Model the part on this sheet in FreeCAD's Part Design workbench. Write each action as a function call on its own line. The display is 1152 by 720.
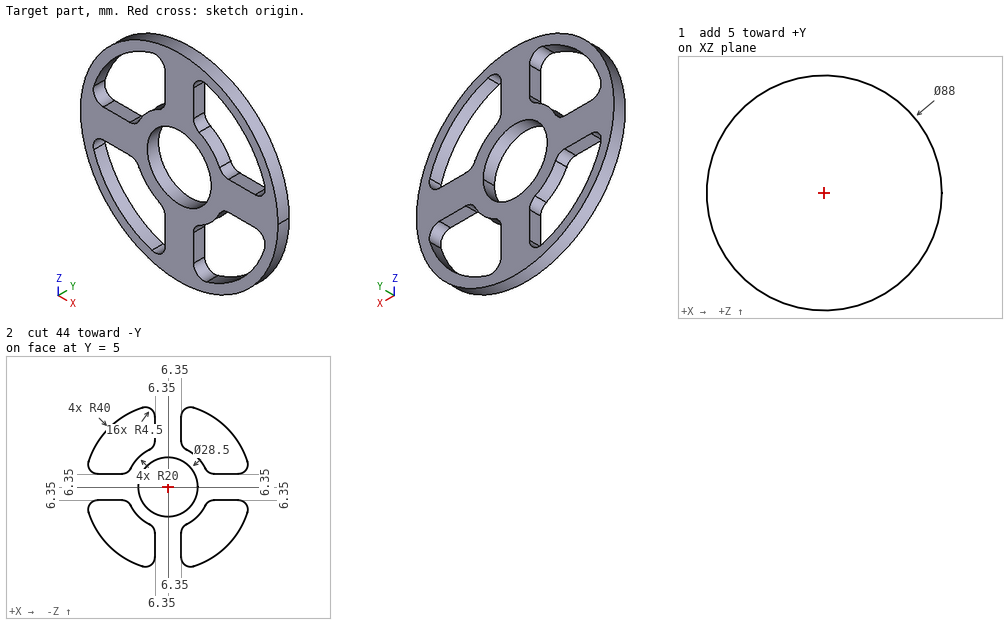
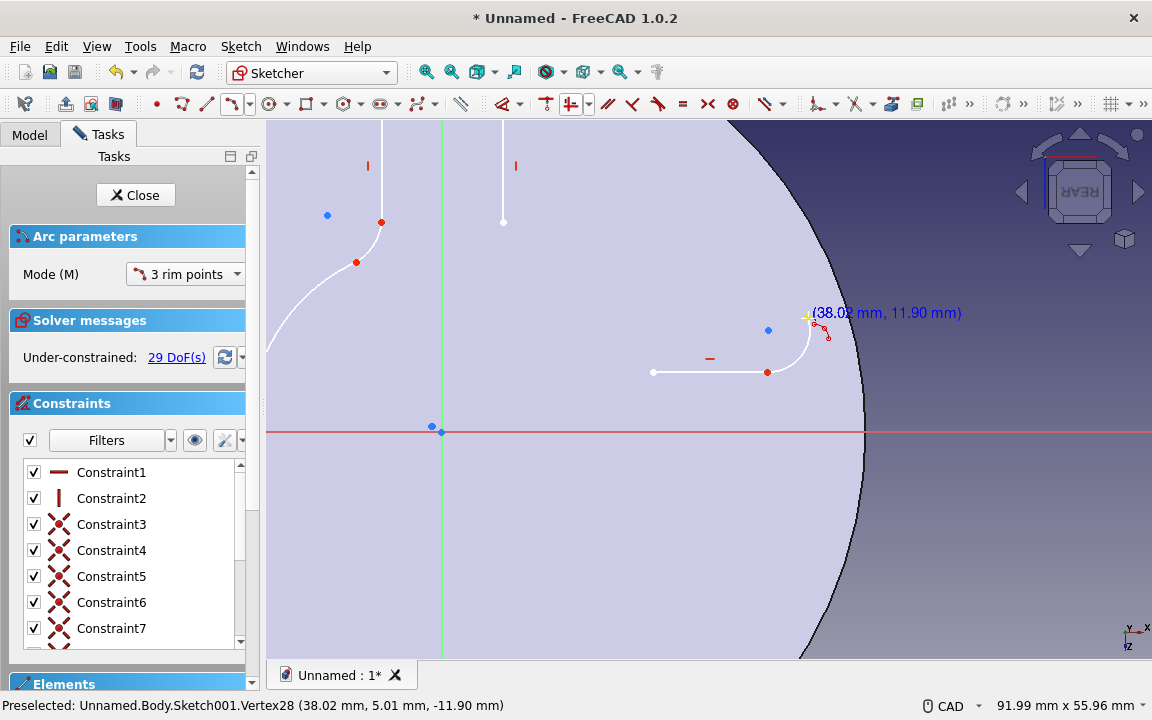
scroll(803, 354, down, 4)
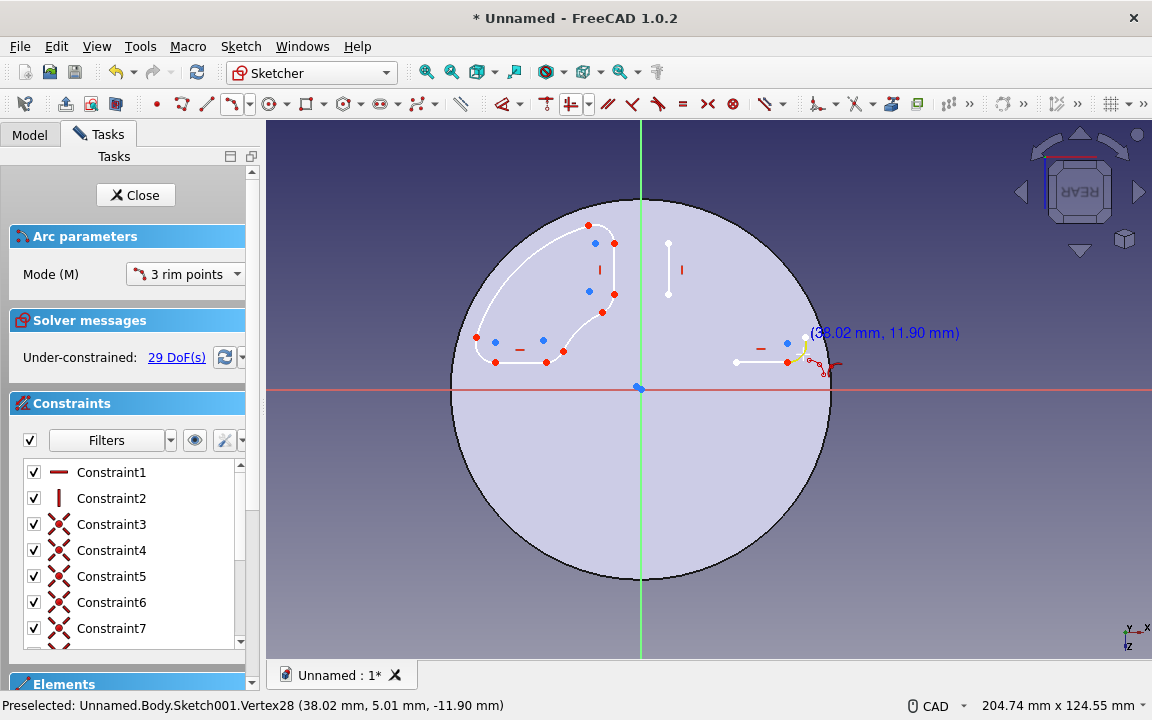
click(694, 225)
click(763, 267)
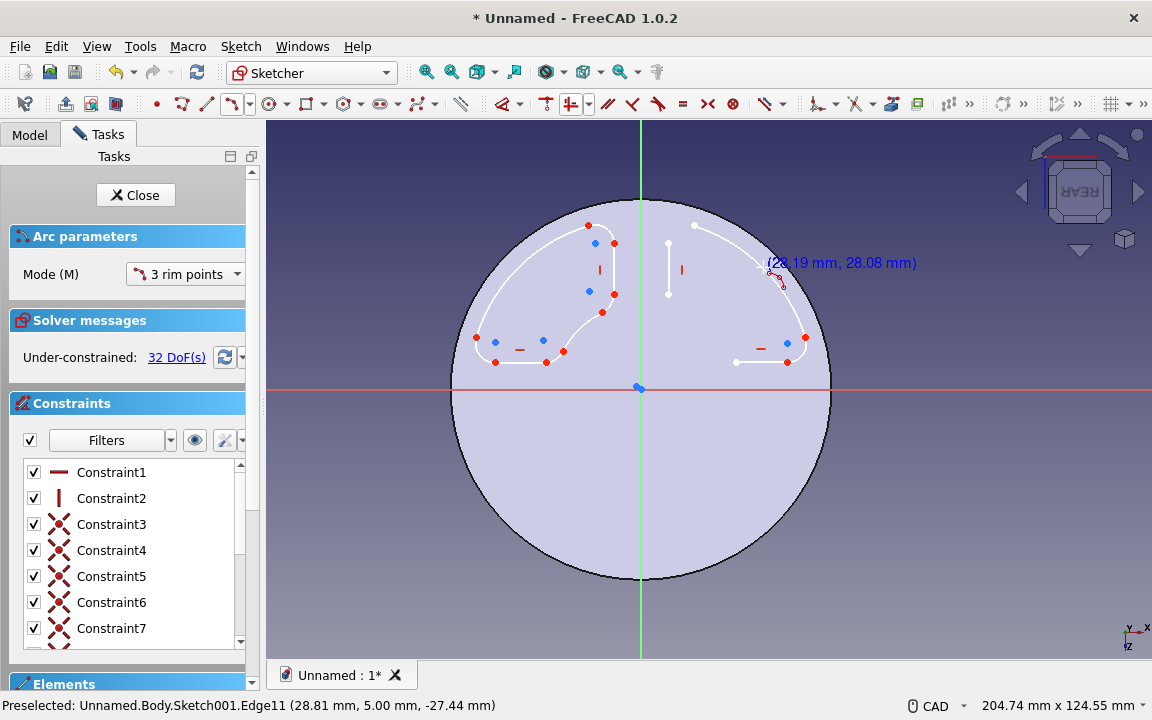
click(694, 226)
click(669, 244)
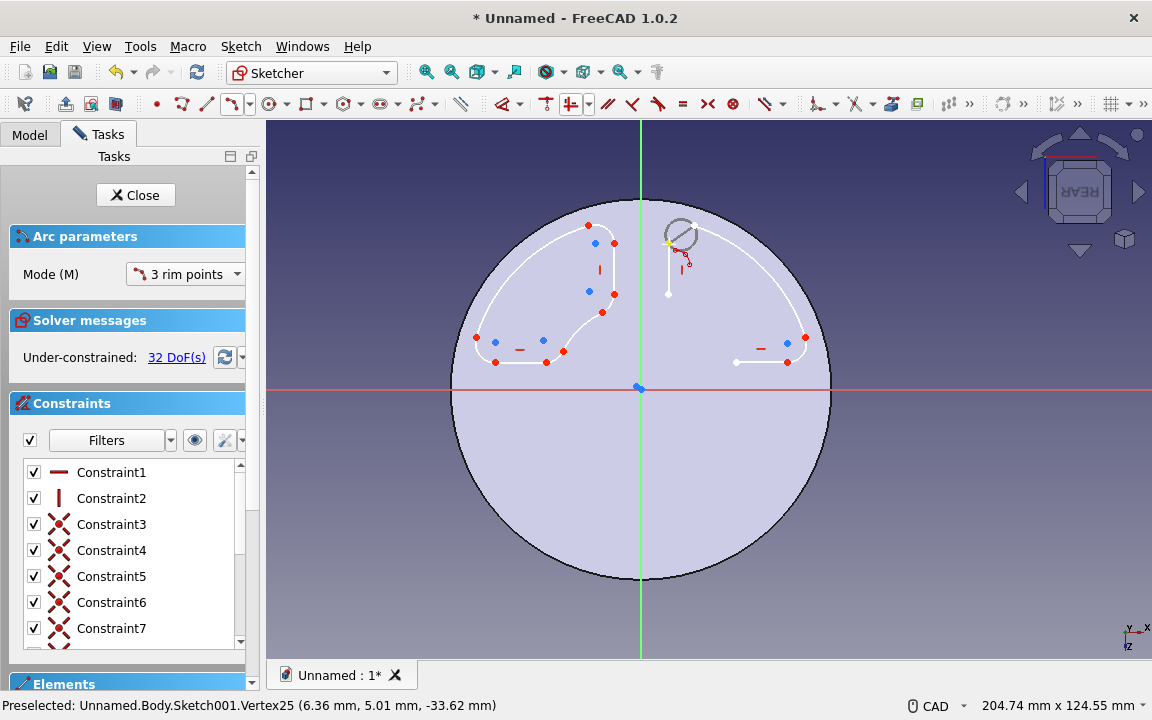
scroll(677, 227, up, 4)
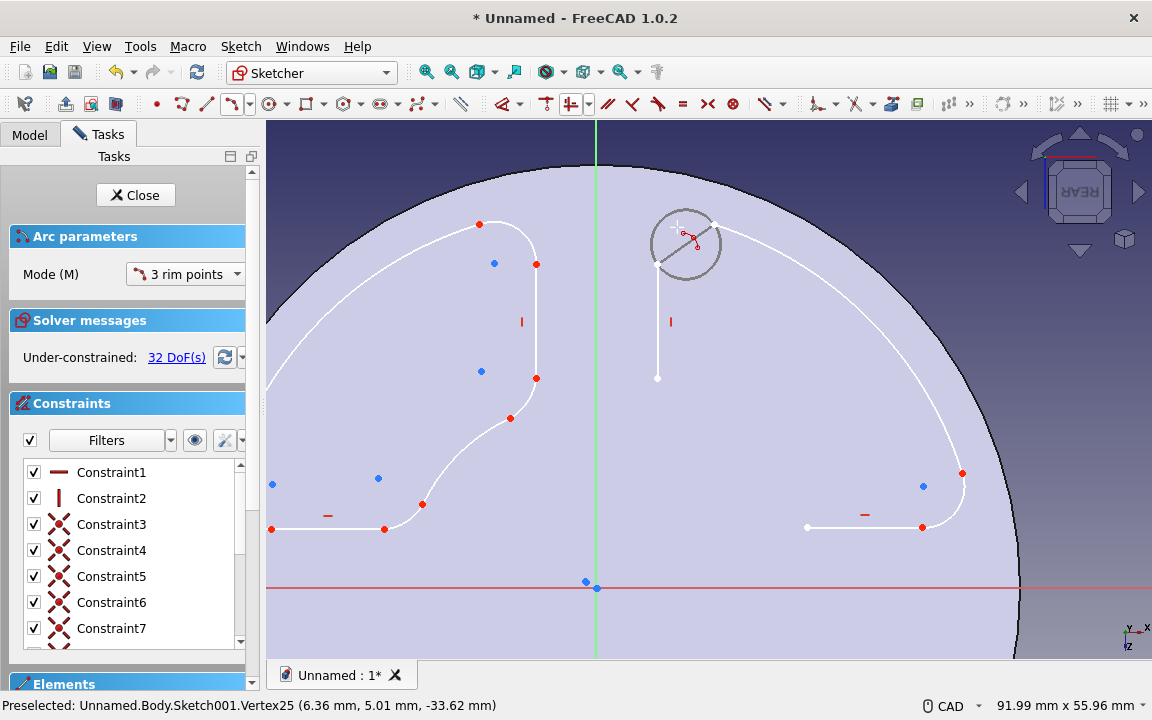
click(675, 228)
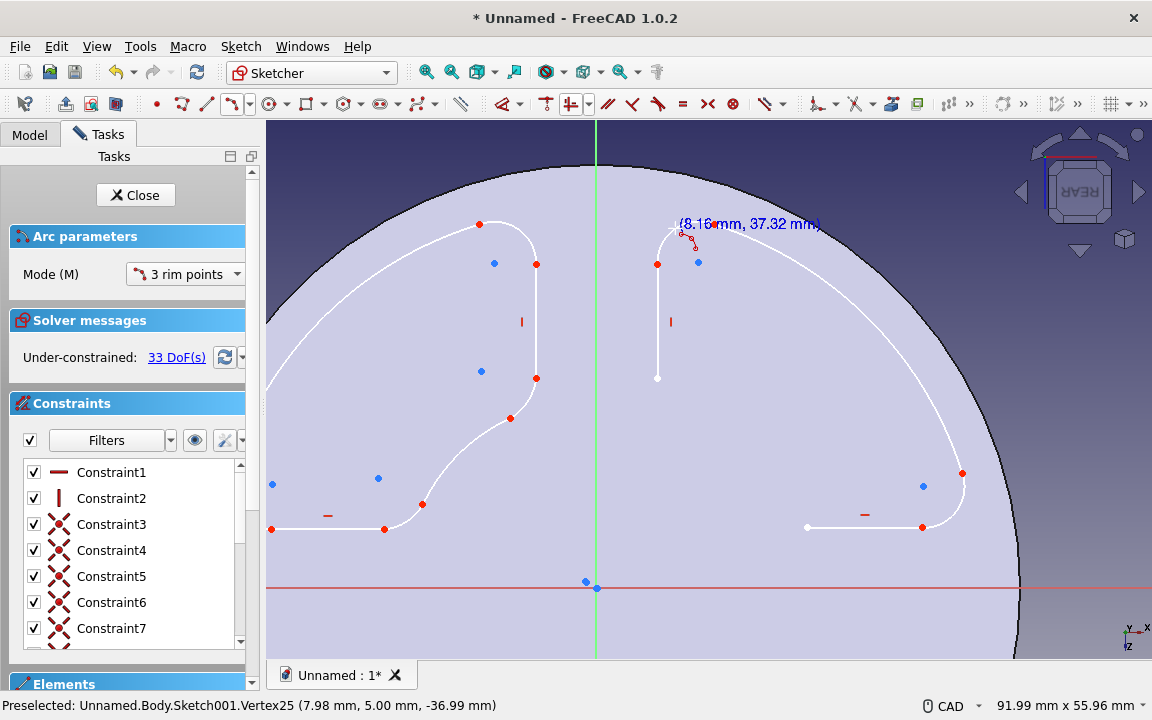
click(658, 378)
click(682, 416)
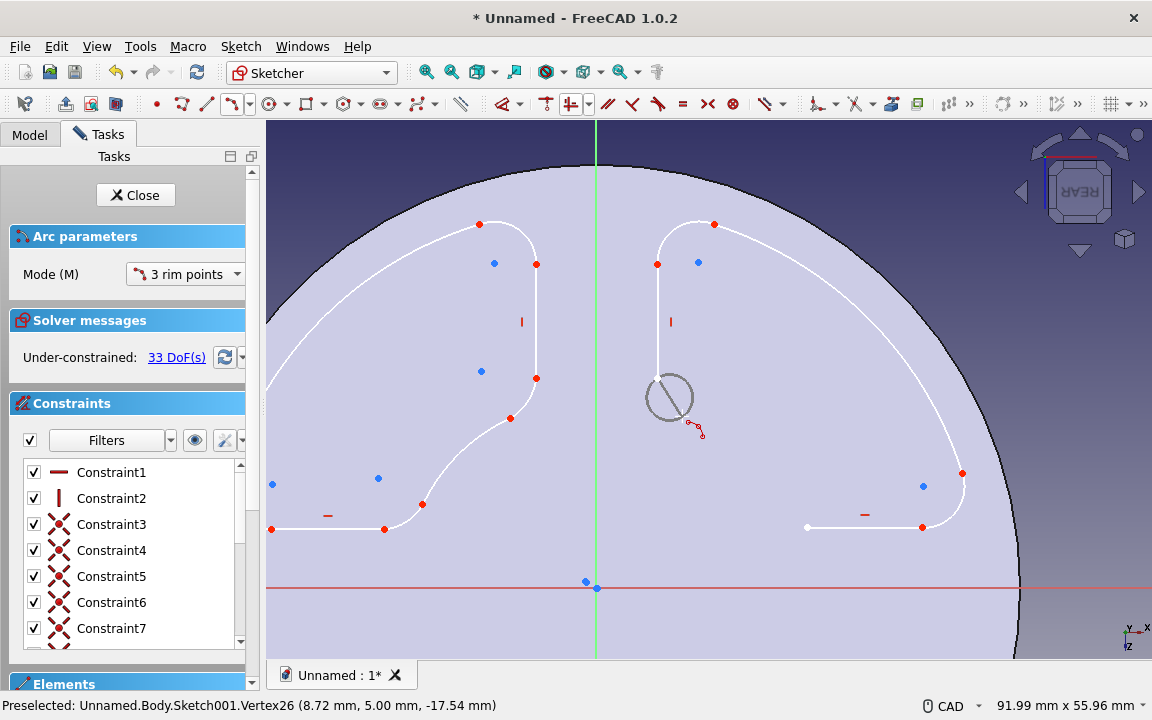
scroll(664, 400, up, 5)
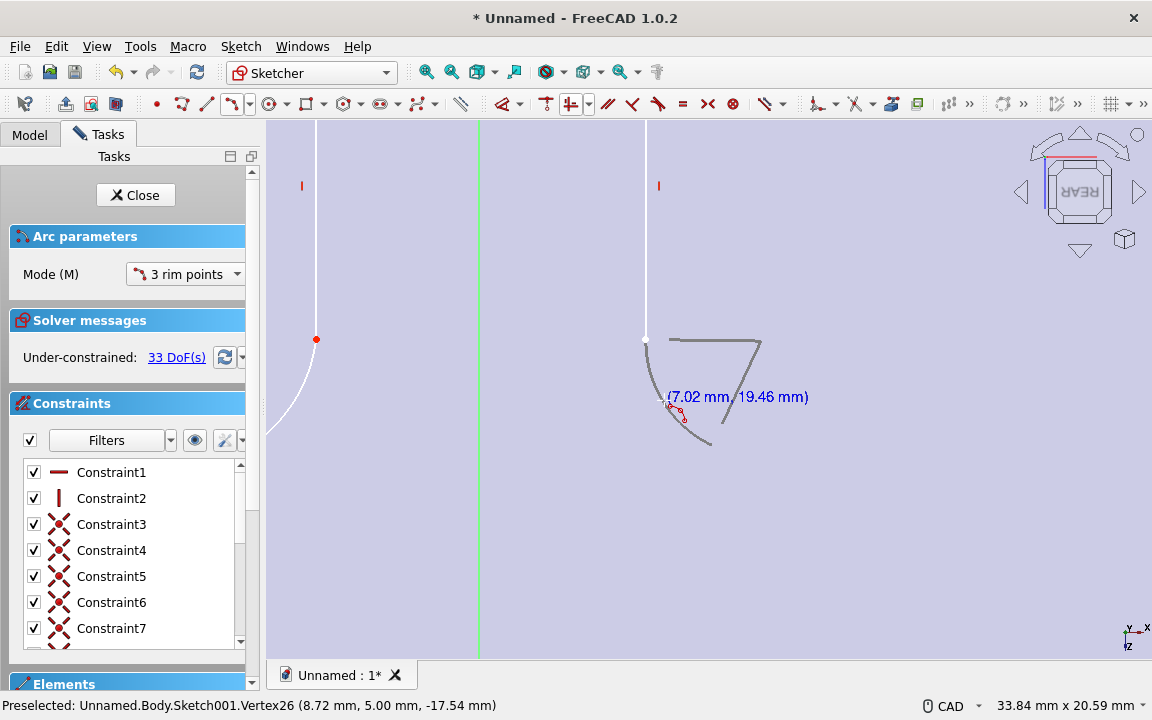
click(663, 398)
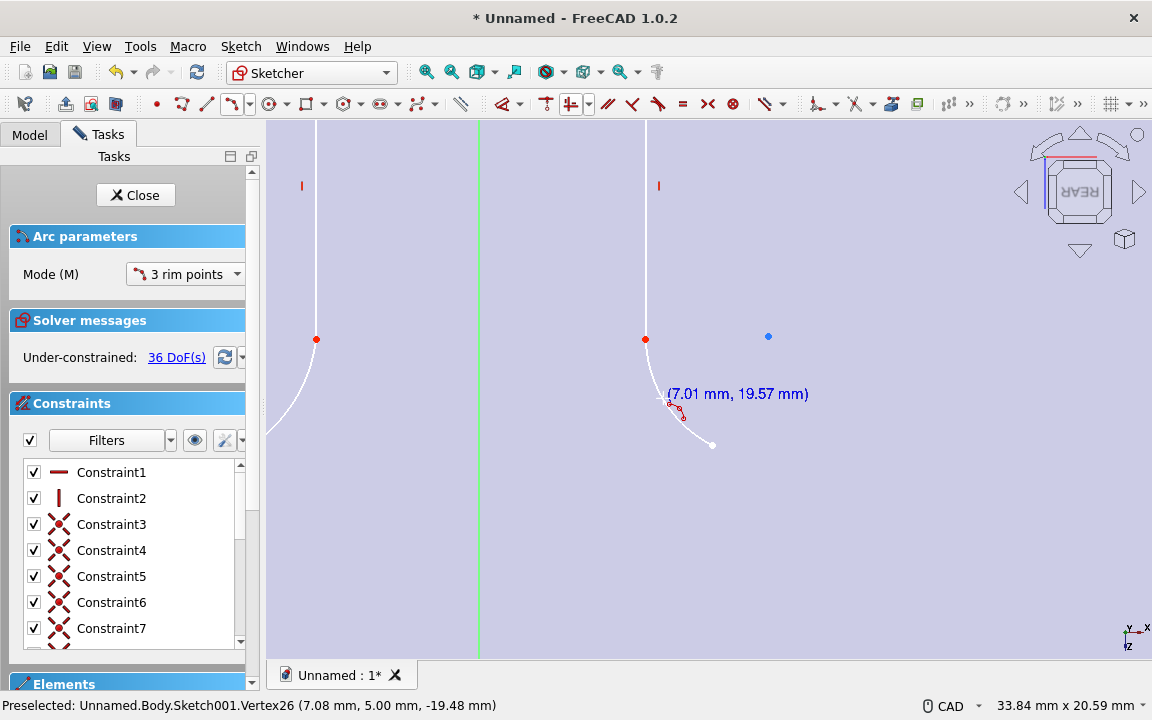
scroll(672, 286, down, 9)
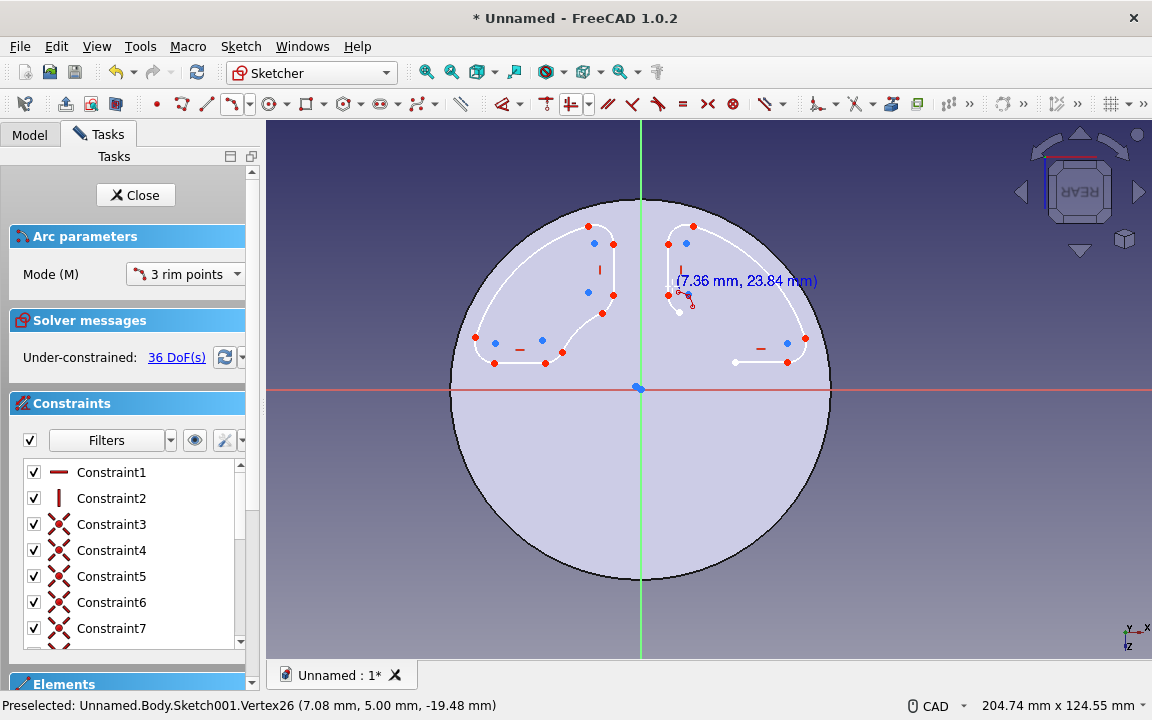
click(679, 313)
click(718, 351)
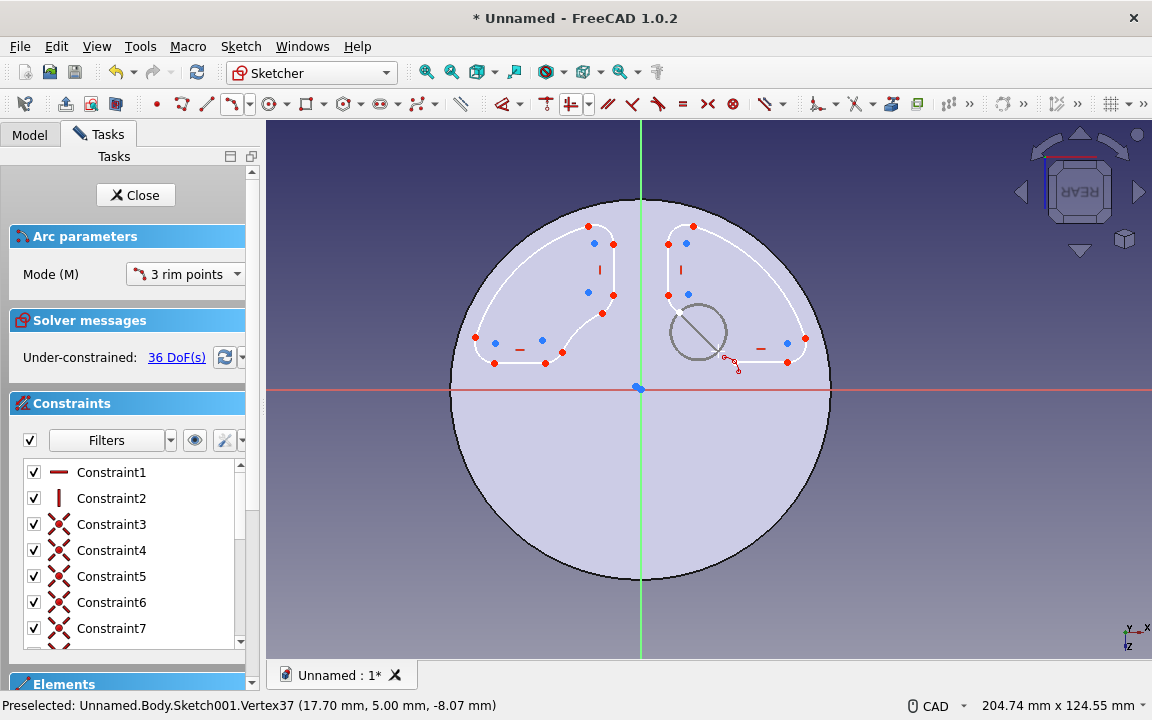
scroll(702, 328, up, 7)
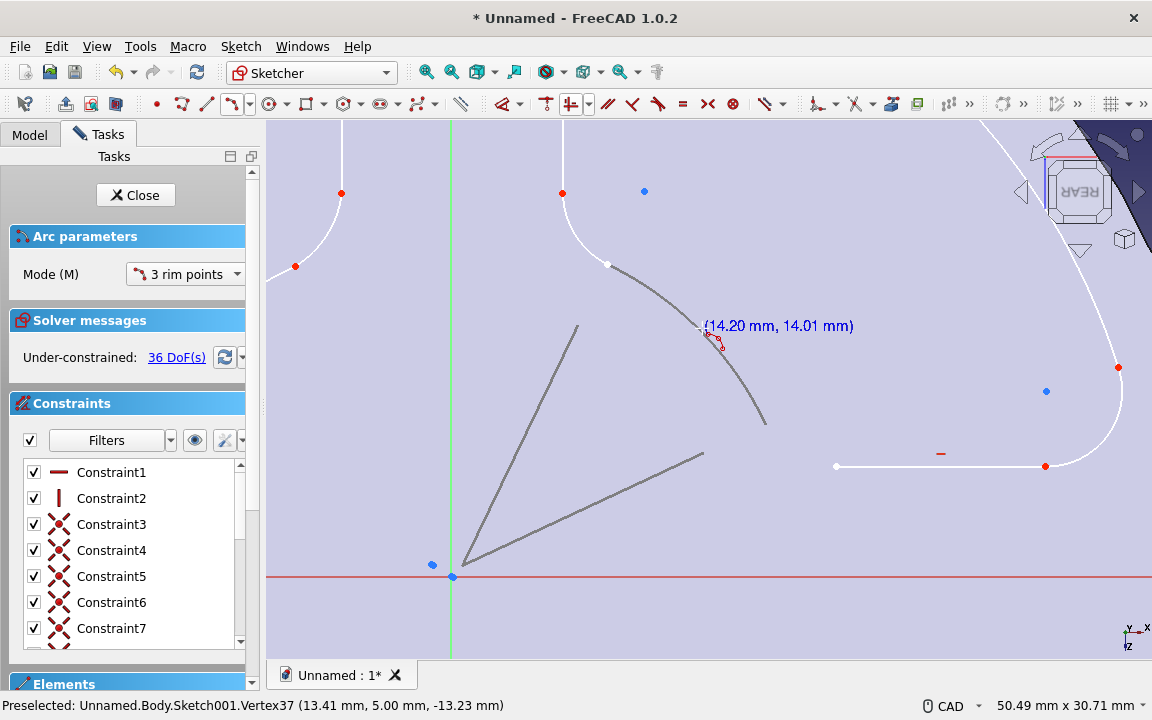
click(699, 328)